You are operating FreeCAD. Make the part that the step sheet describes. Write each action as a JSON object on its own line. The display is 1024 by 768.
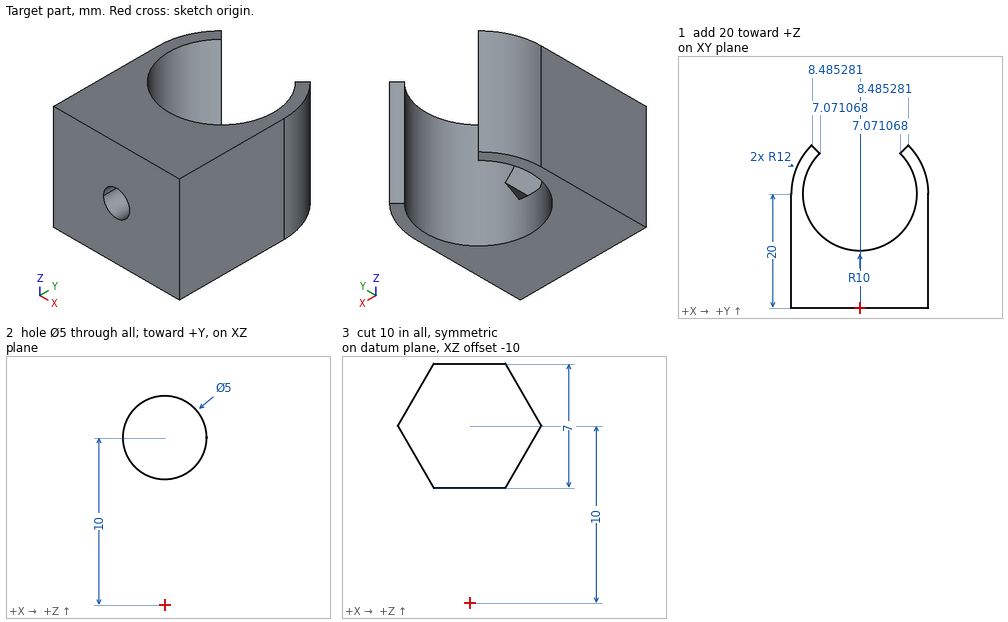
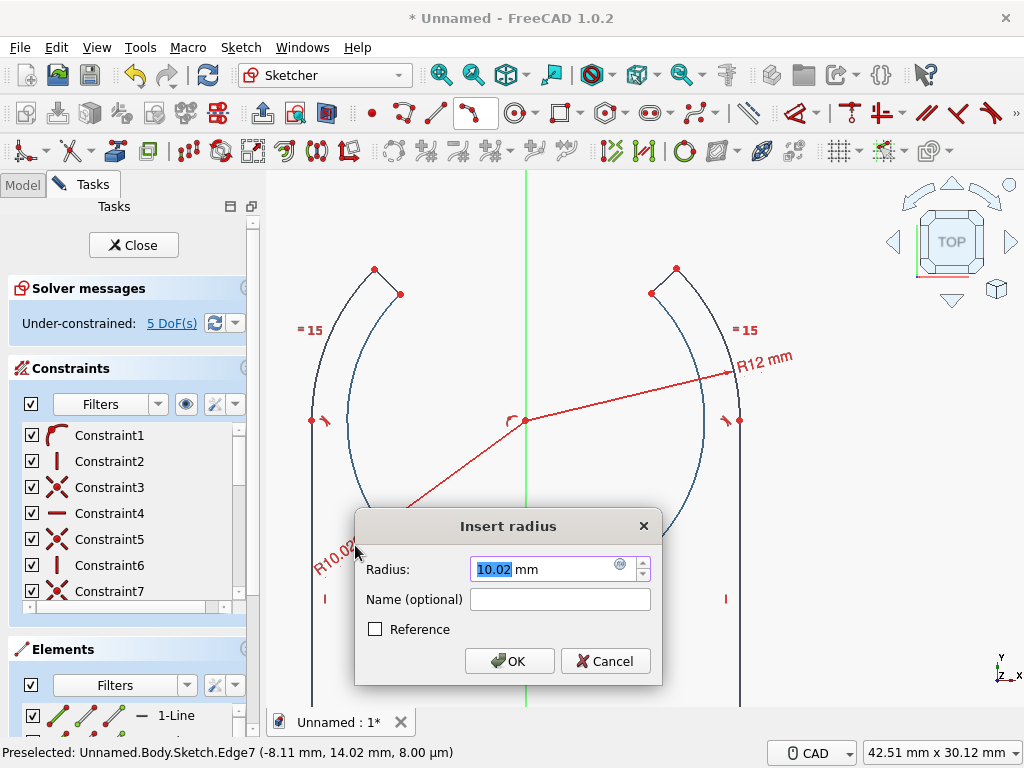
{"action": "type", "text": "10"}
{"action": "key", "text": "Return"}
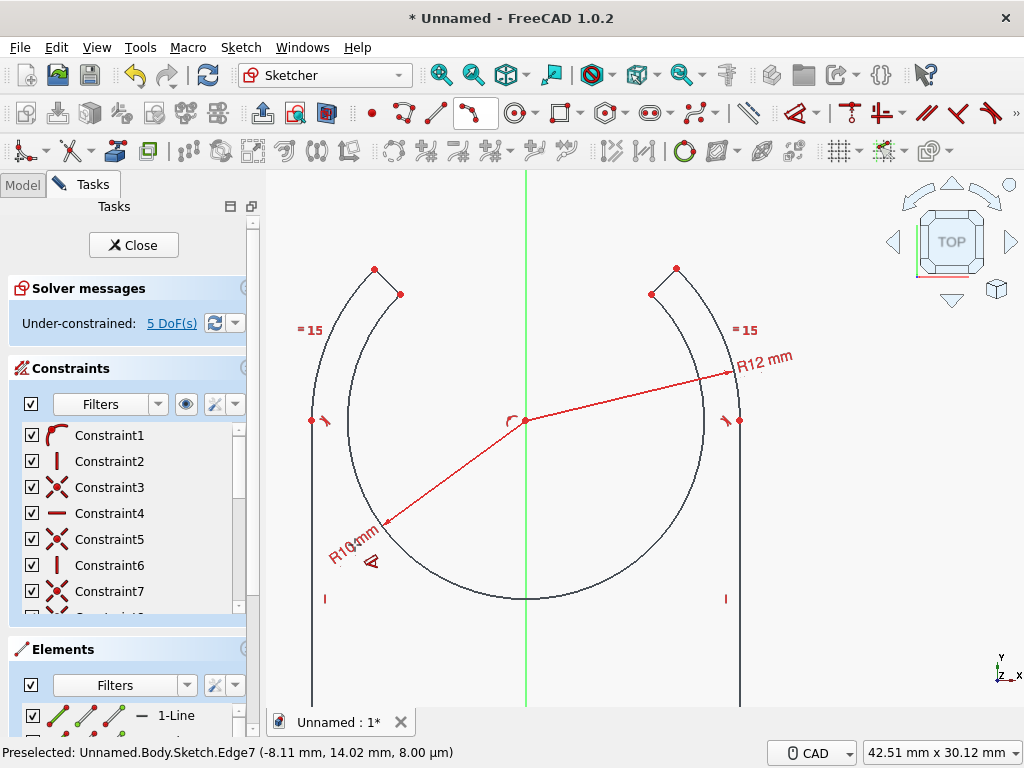
{"action": "left_click", "coordinate": [312, 527]}
{"action": "left_click", "coordinate": [346, 491]}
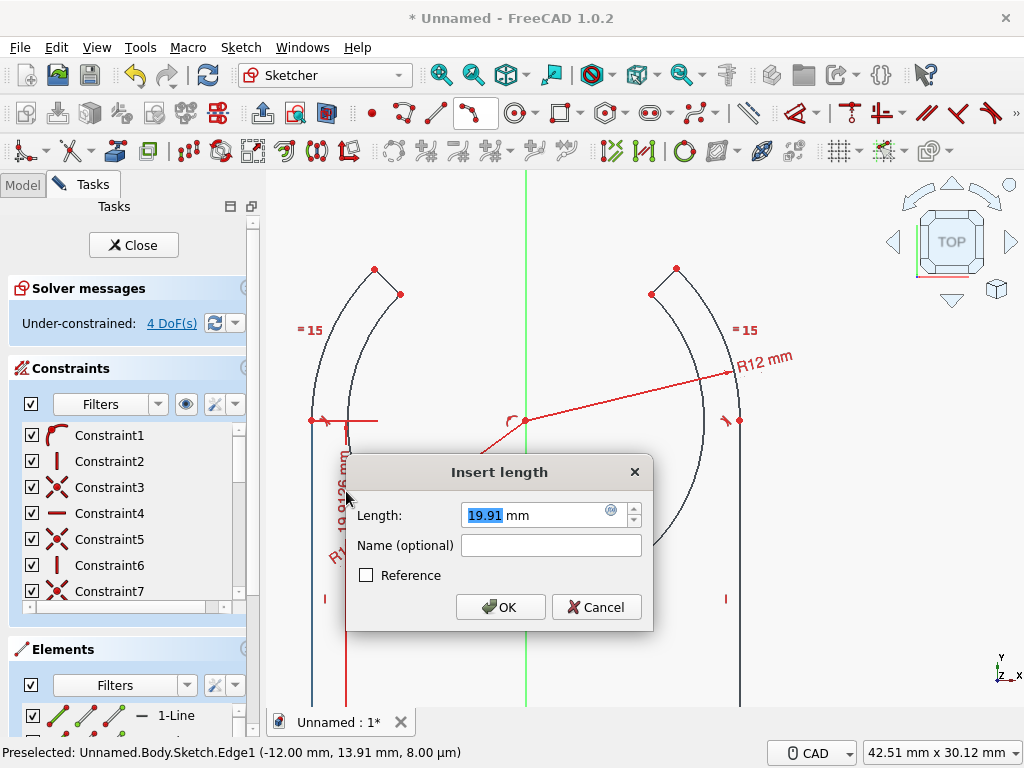
{"action": "type", "text": "20"}
{"action": "key", "text": "Return"}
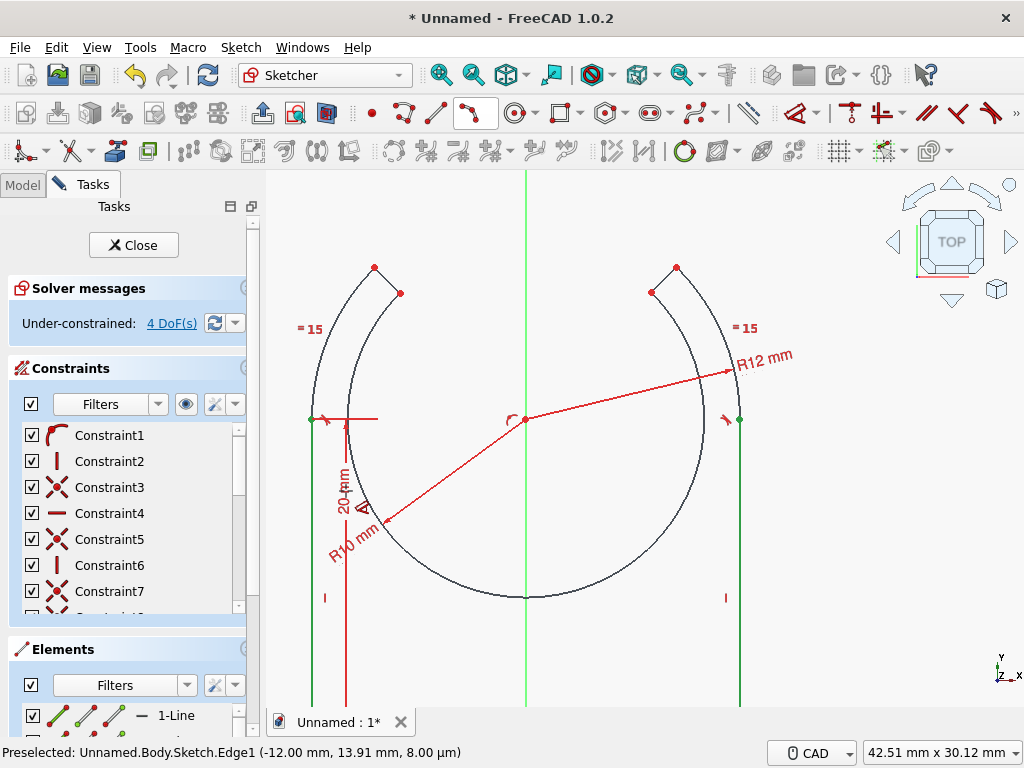
{"action": "left_click", "coordinate": [676, 267]}
{"action": "left_click", "coordinate": [601, 233]}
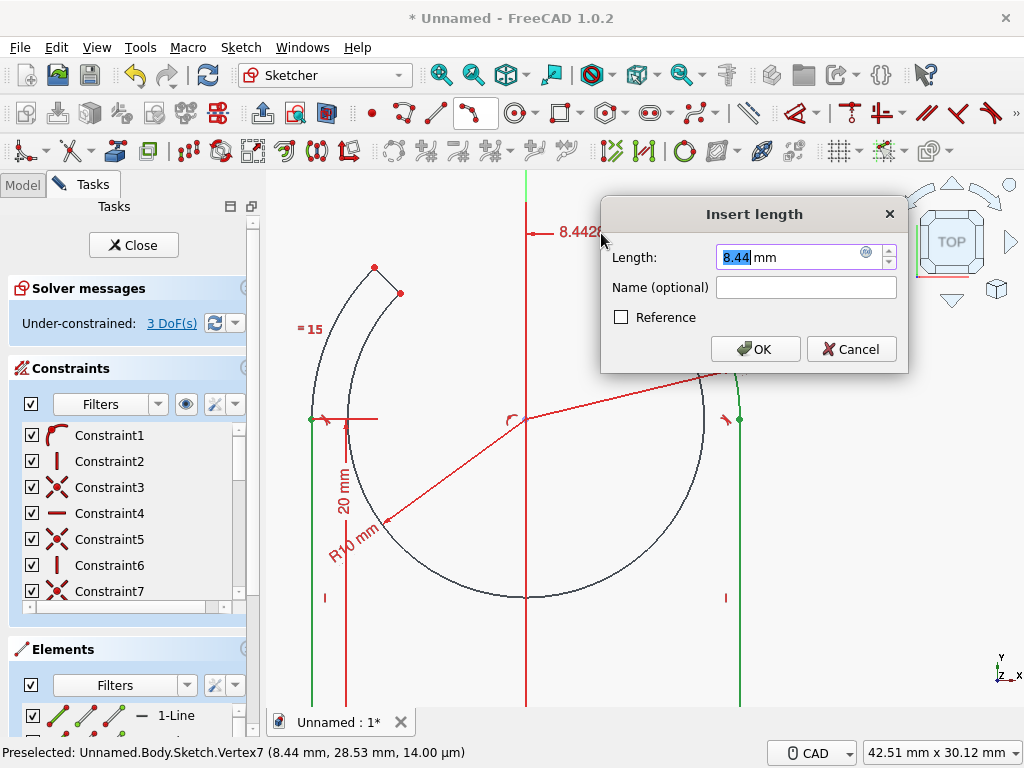
{"action": "type", "text": "8.485281"}
{"action": "key", "text": "Return"}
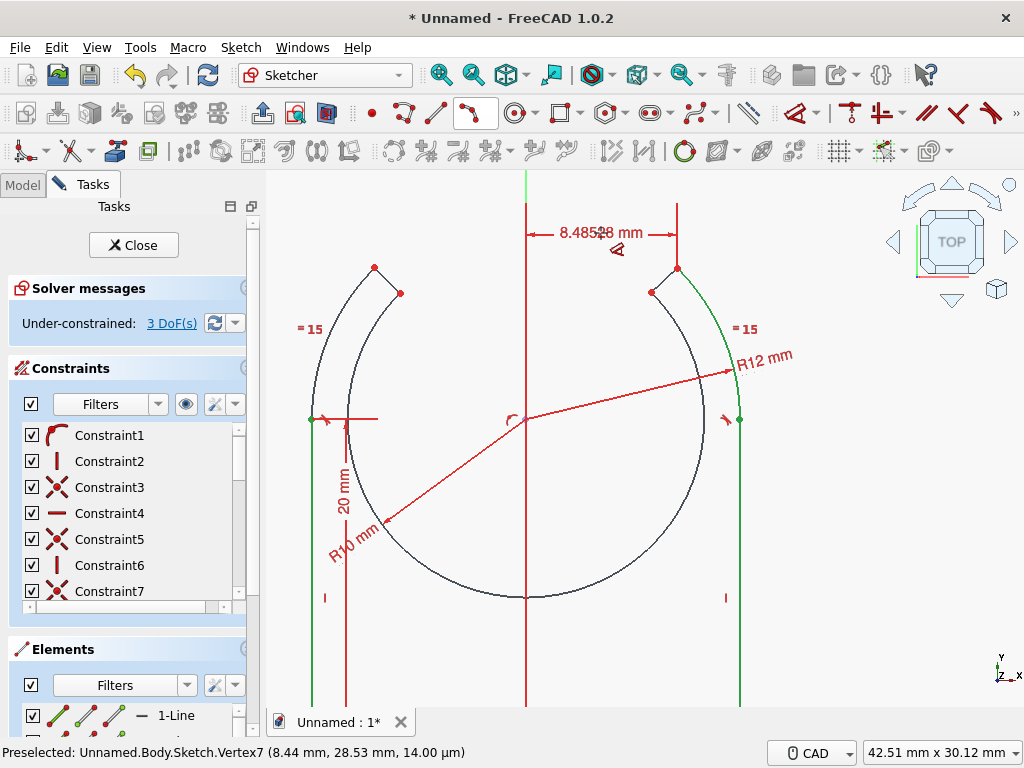
{"action": "left_click", "coordinate": [651, 292]}
{"action": "left_click", "coordinate": [589, 258]}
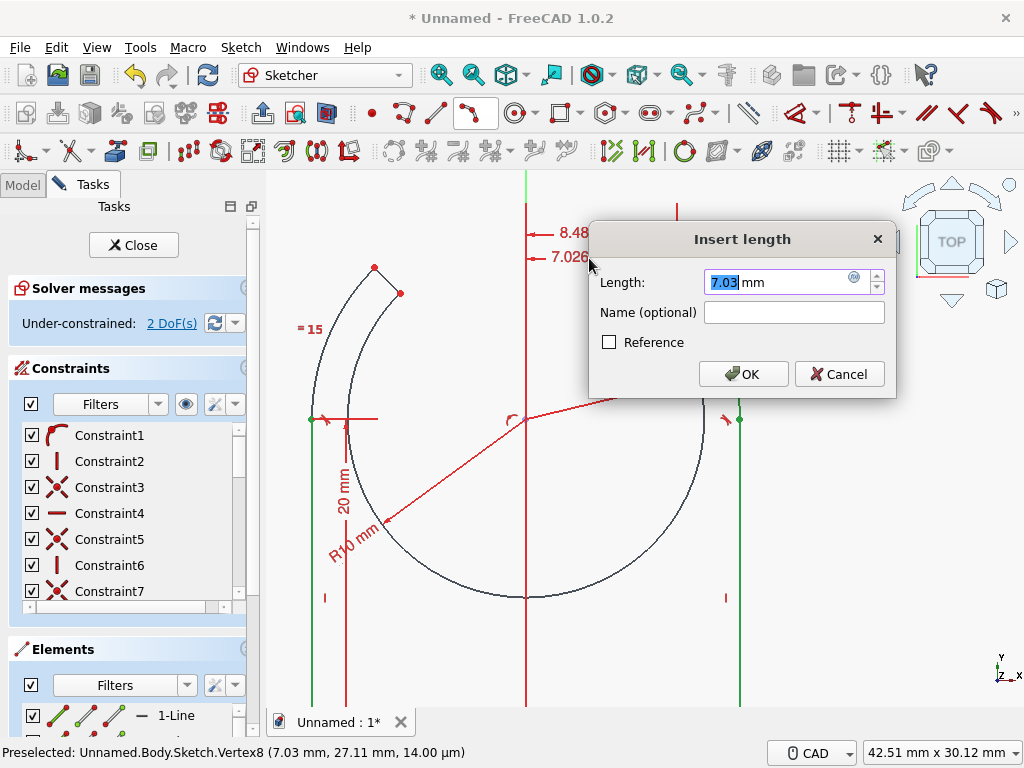
{"action": "type", "text": "7.071068"}
{"action": "key", "text": "Return"}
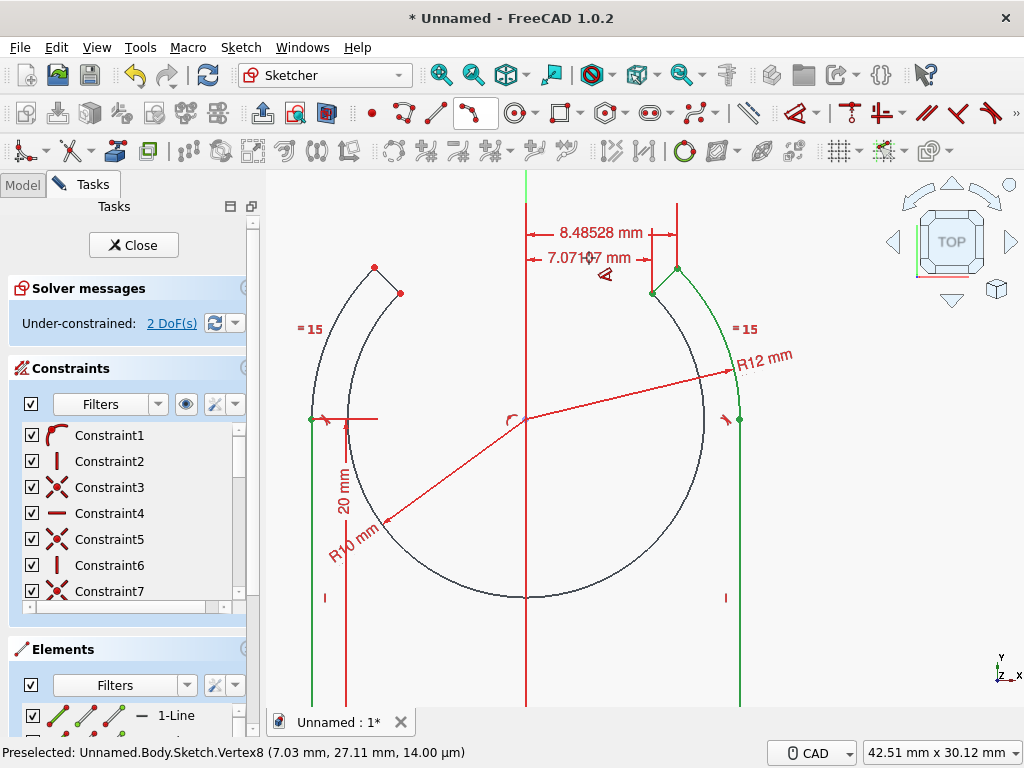
{"action": "left_click", "coordinate": [400, 293]}
{"action": "left_click", "coordinate": [463, 259]}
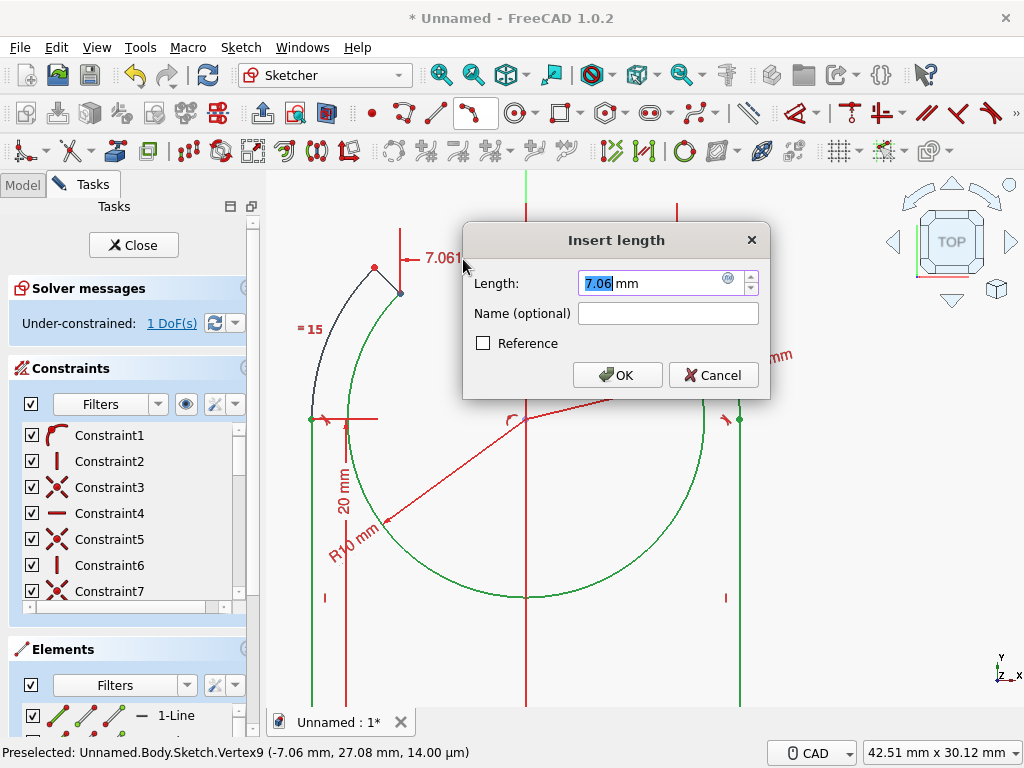
{"action": "type", "text": "7.071068"}
{"action": "key", "text": "Return"}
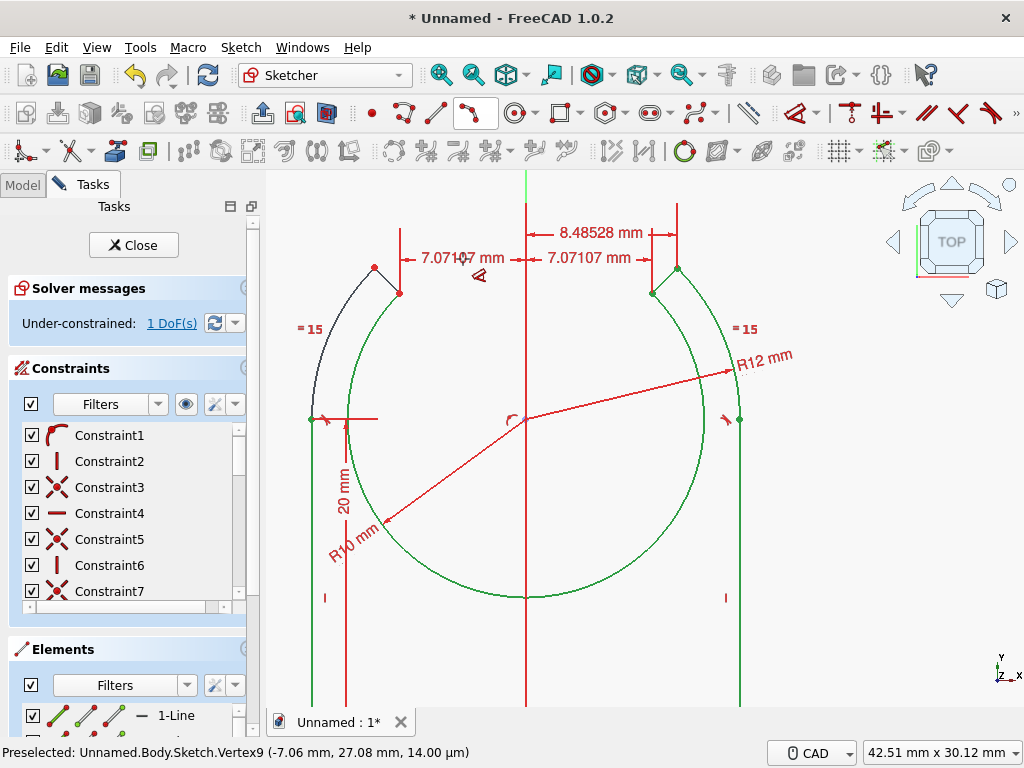
{"action": "left_click", "coordinate": [375, 268]}
{"action": "left_click", "coordinate": [450, 234]}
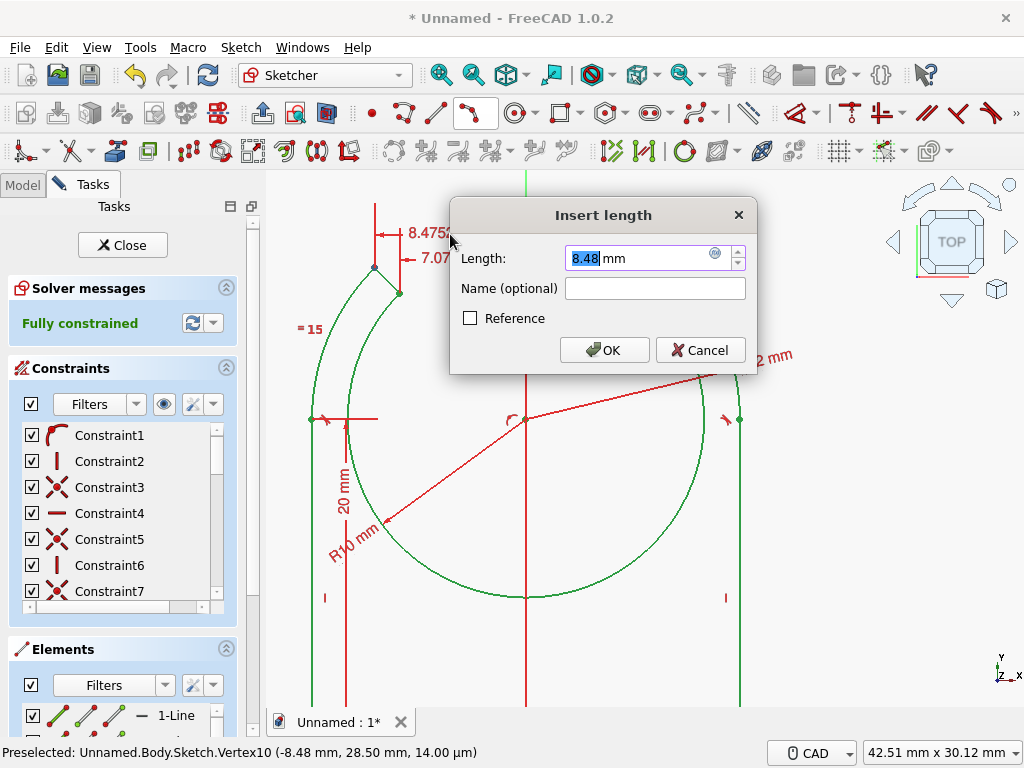
{"action": "type", "text": "8.485281"}
{"action": "key", "text": "Return"}
{"action": "key", "text": "Escape"}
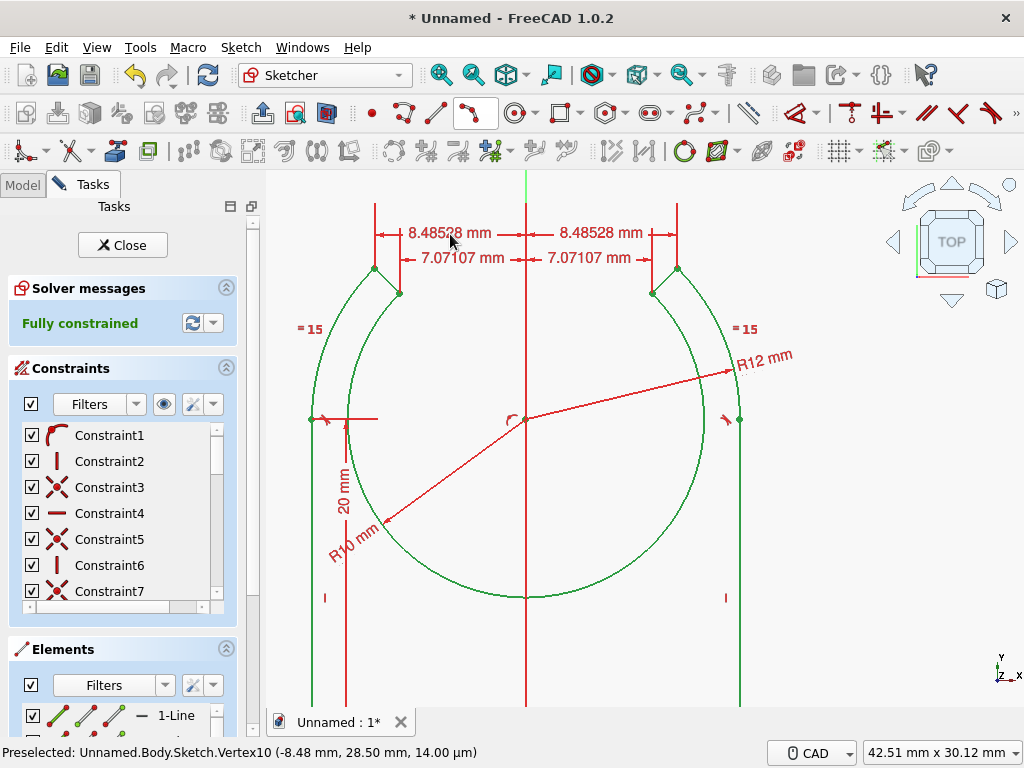
{"action": "left_click", "coordinate": [123, 245]}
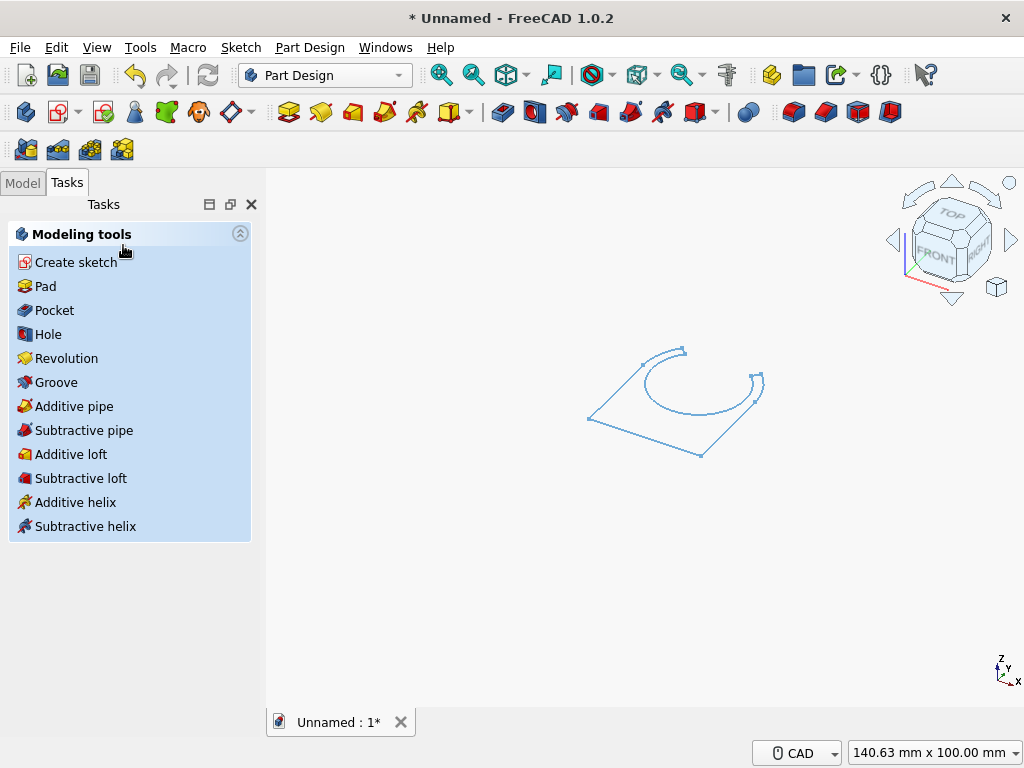
{"action": "left_click", "coordinate": [290, 112]}